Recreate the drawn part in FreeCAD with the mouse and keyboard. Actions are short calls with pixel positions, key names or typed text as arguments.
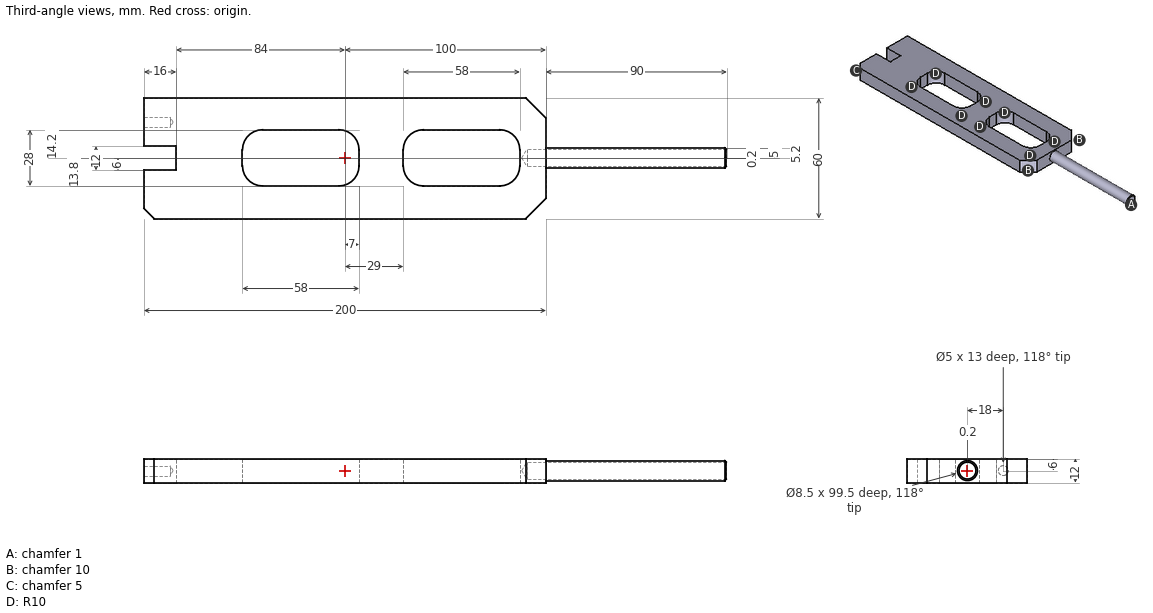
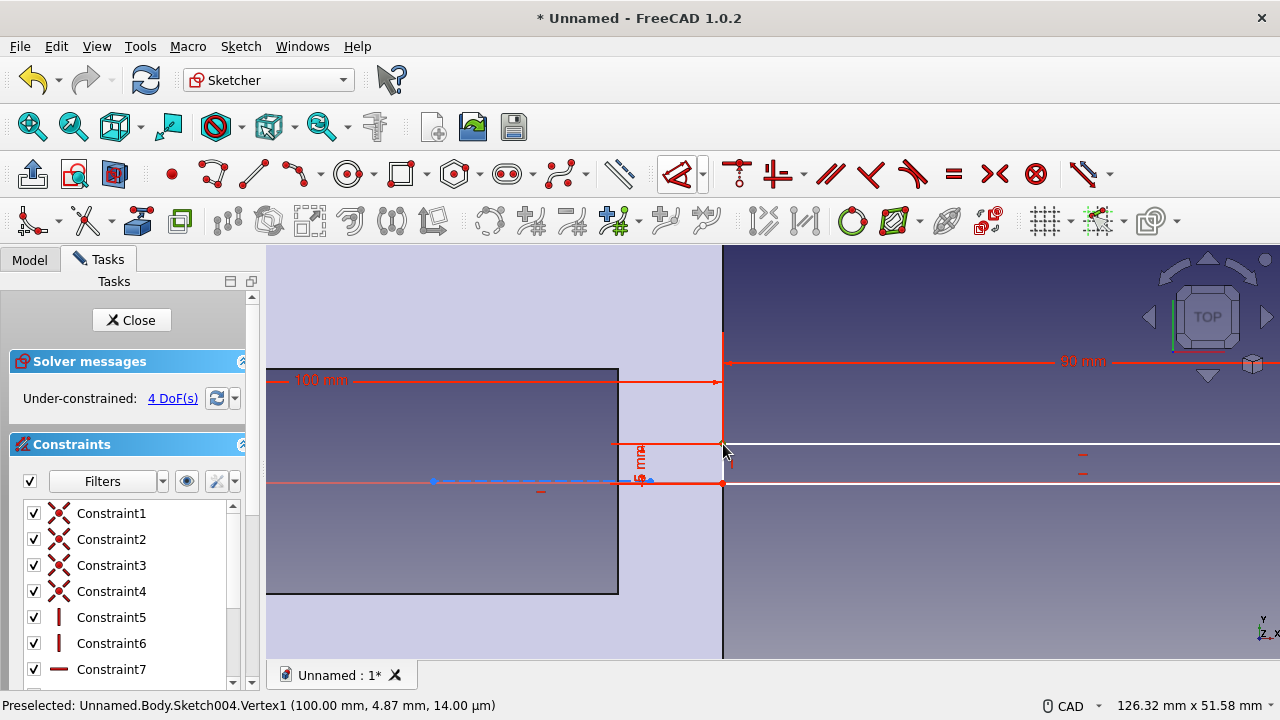
key(i)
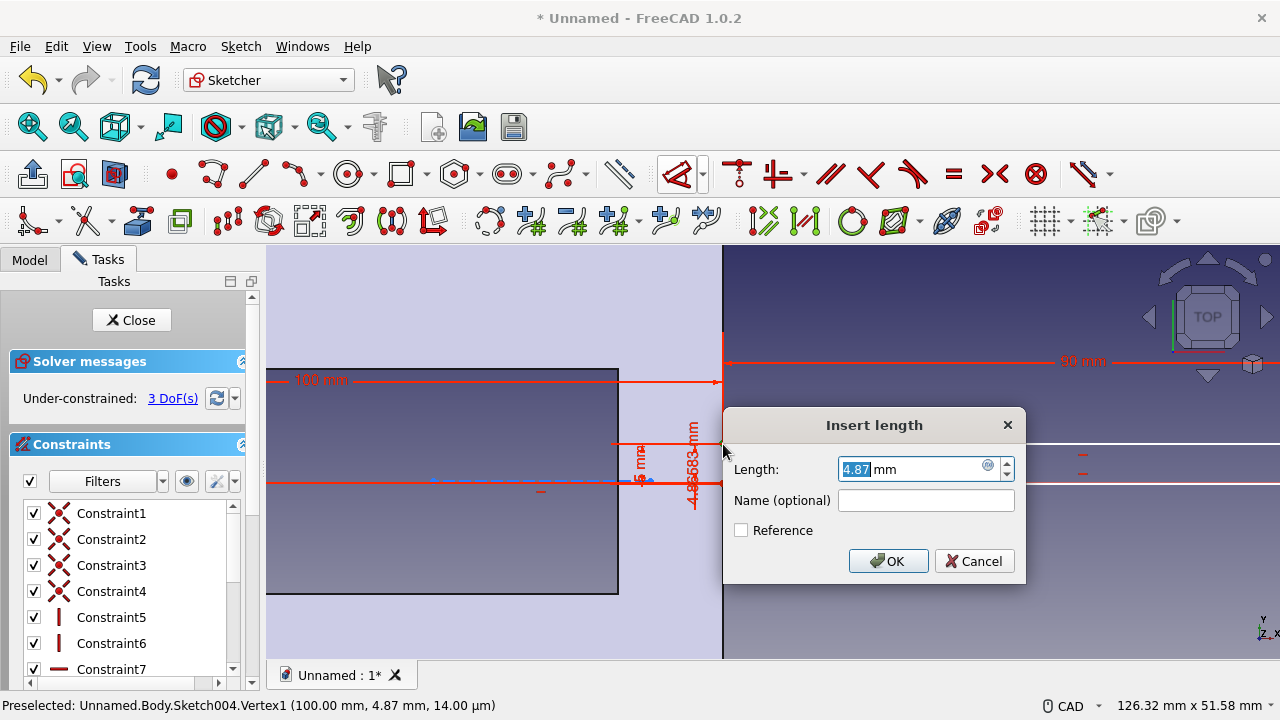
text(5.2)
key(Return)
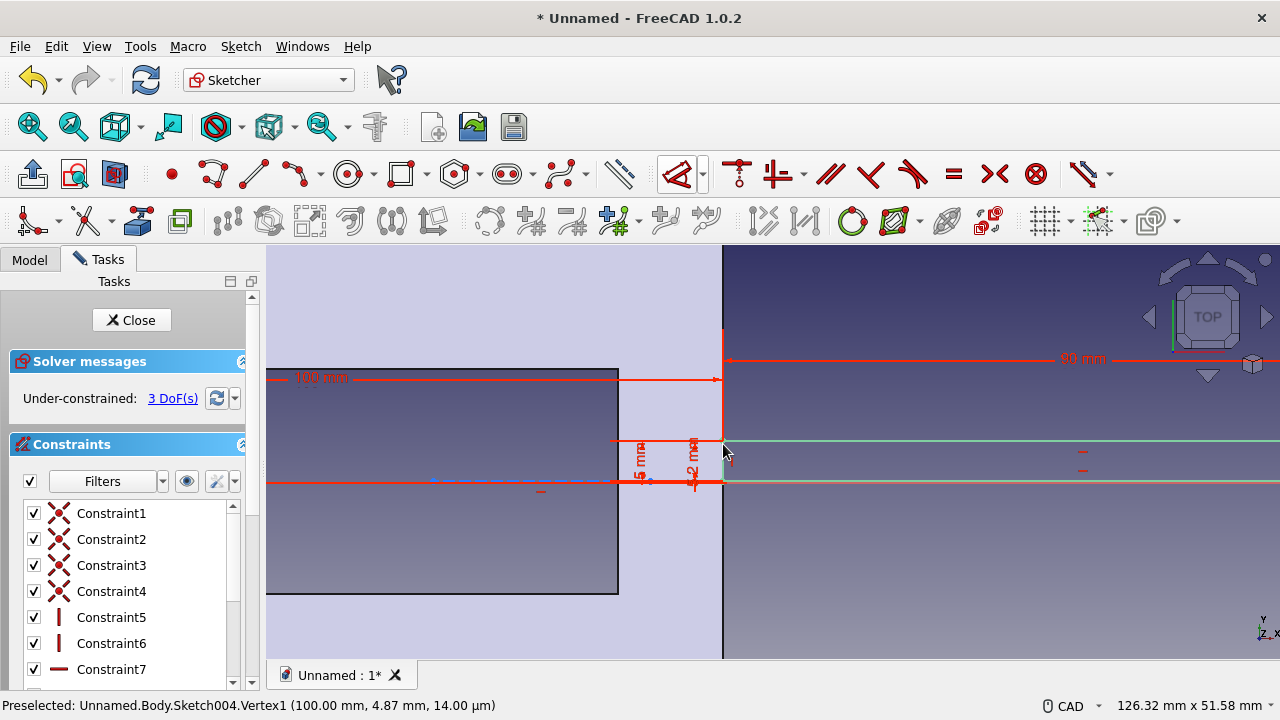
scroll(650, 481, up, 17)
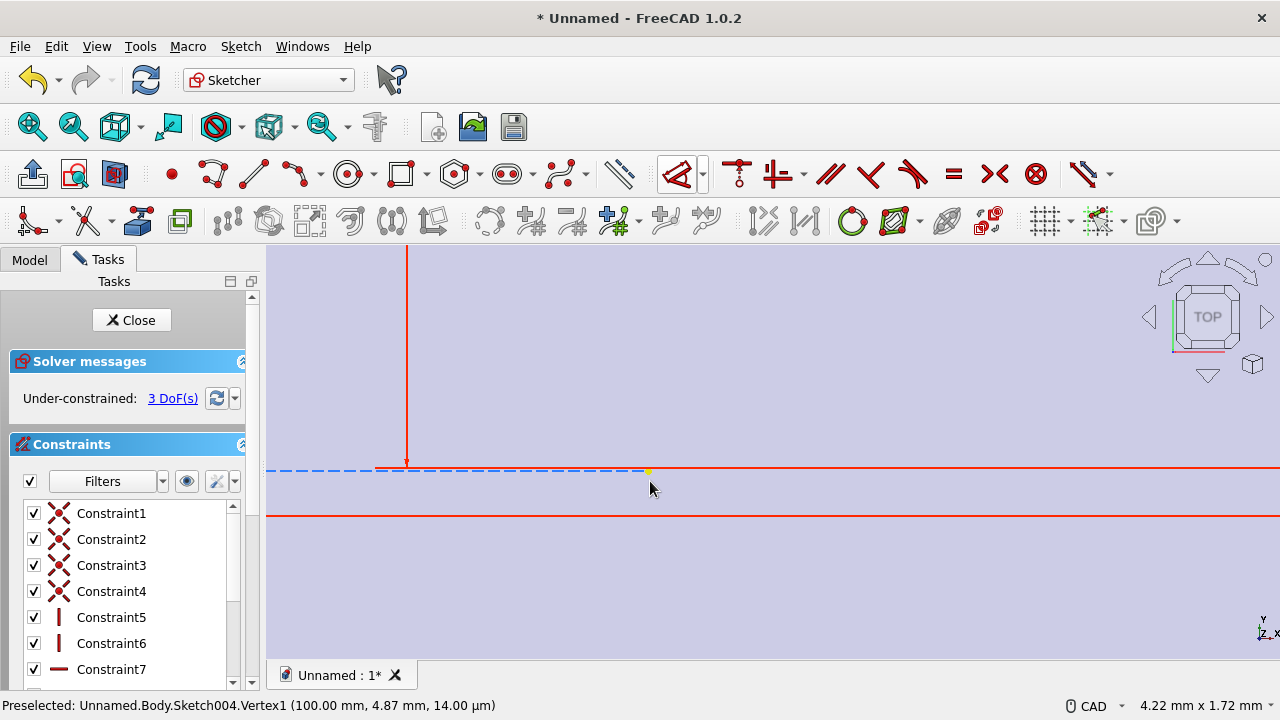
click(648, 471)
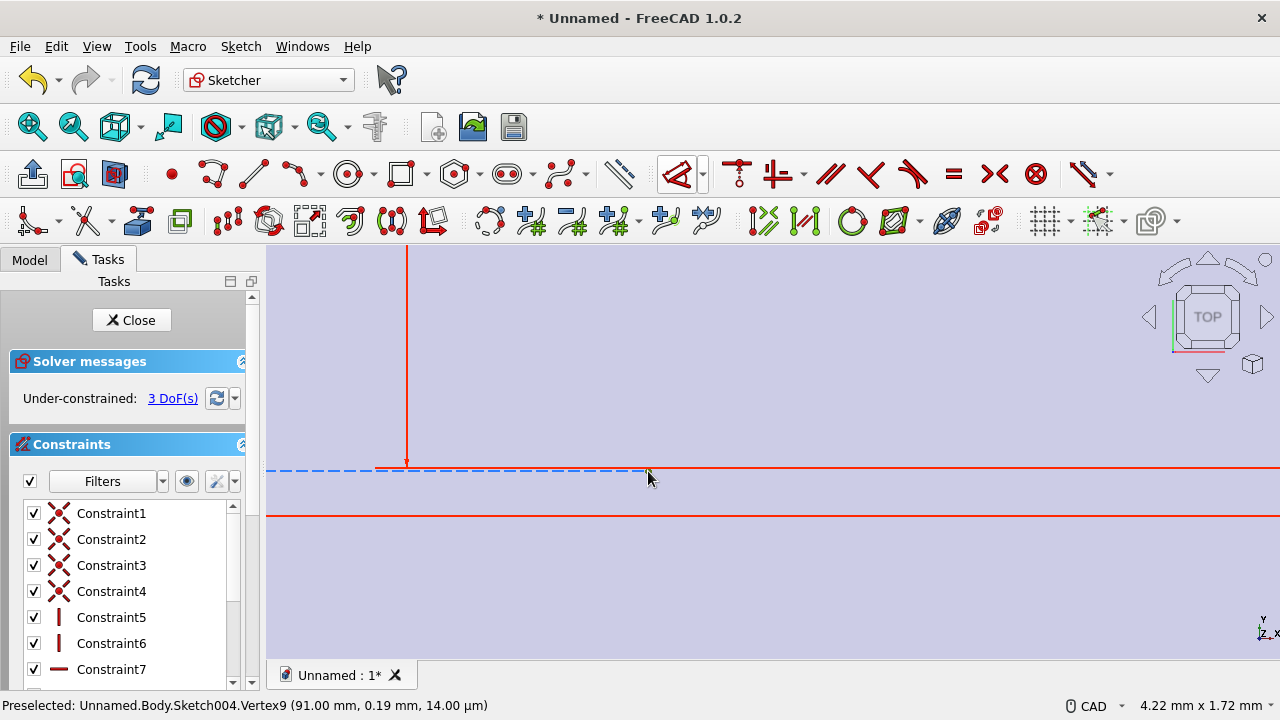
click(702, 174)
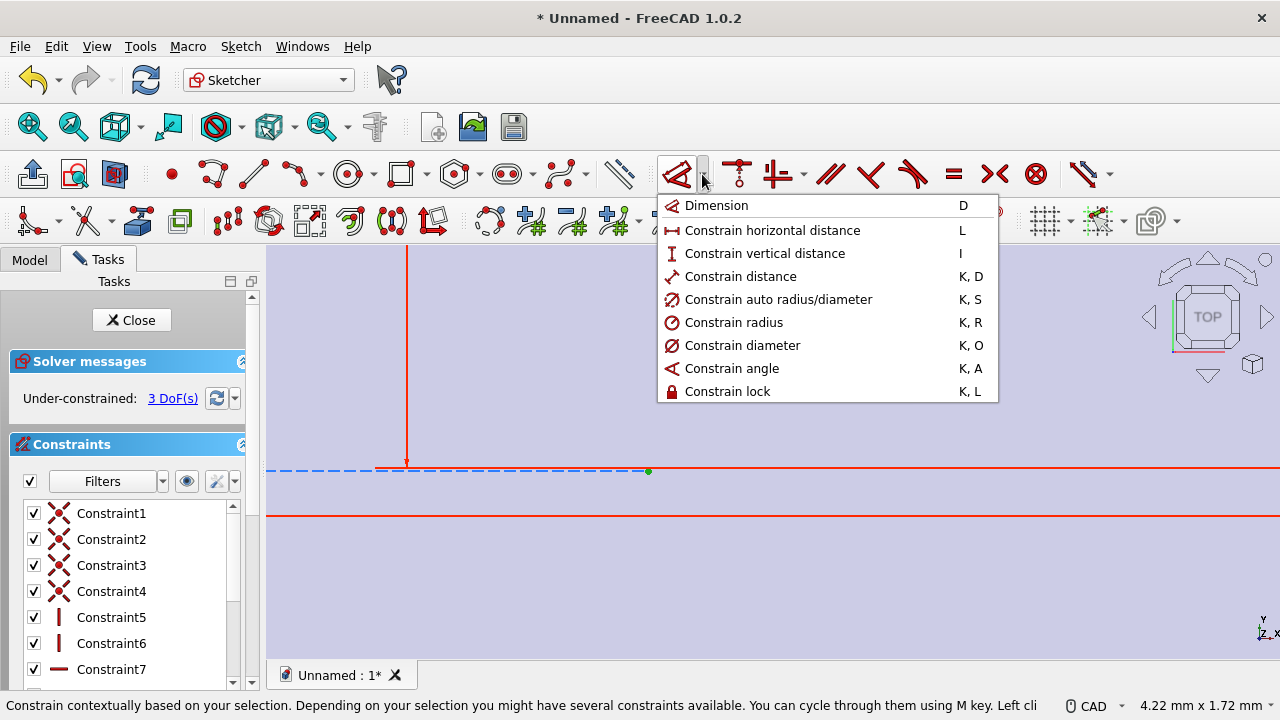
click(828, 254)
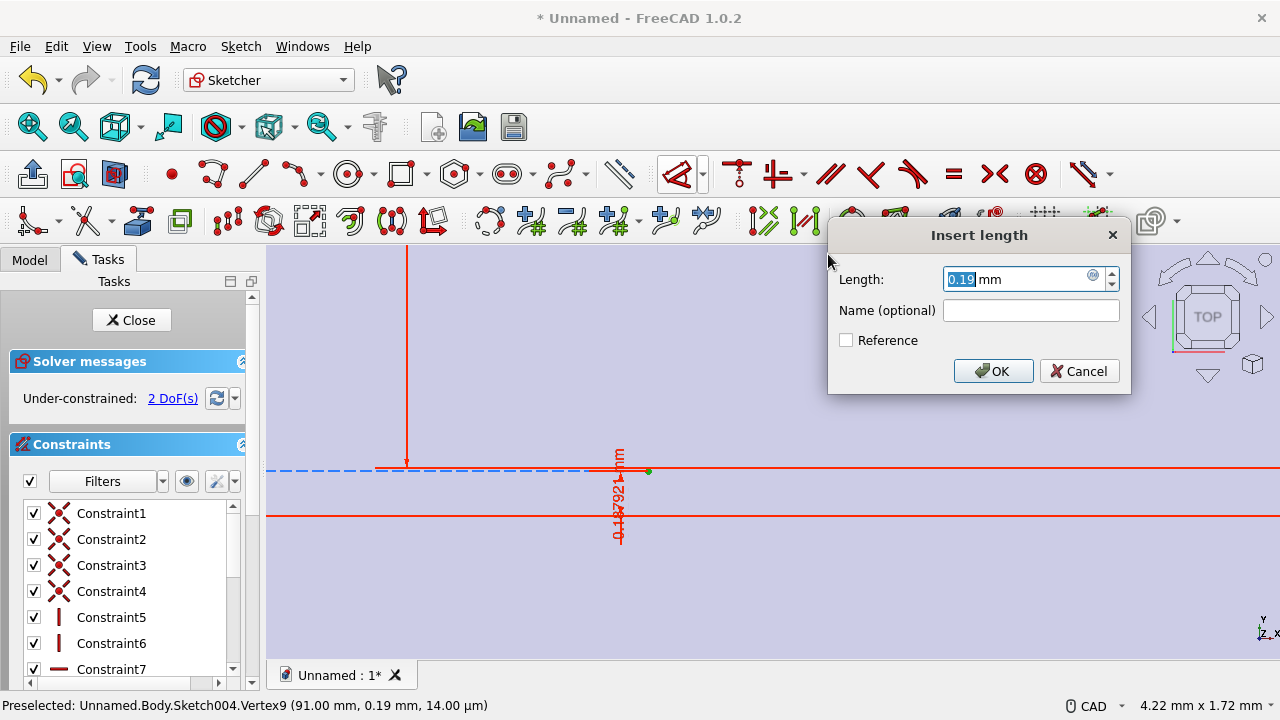
text(0.2)
key(Return)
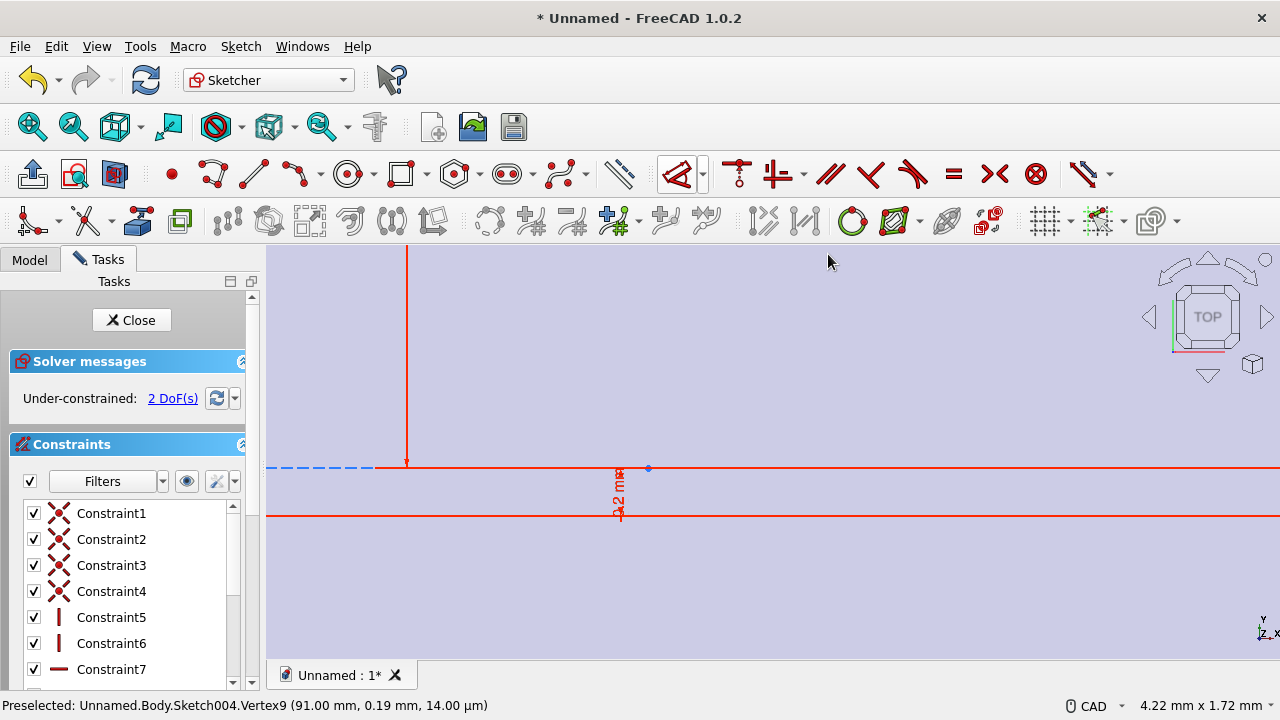
click(132, 320)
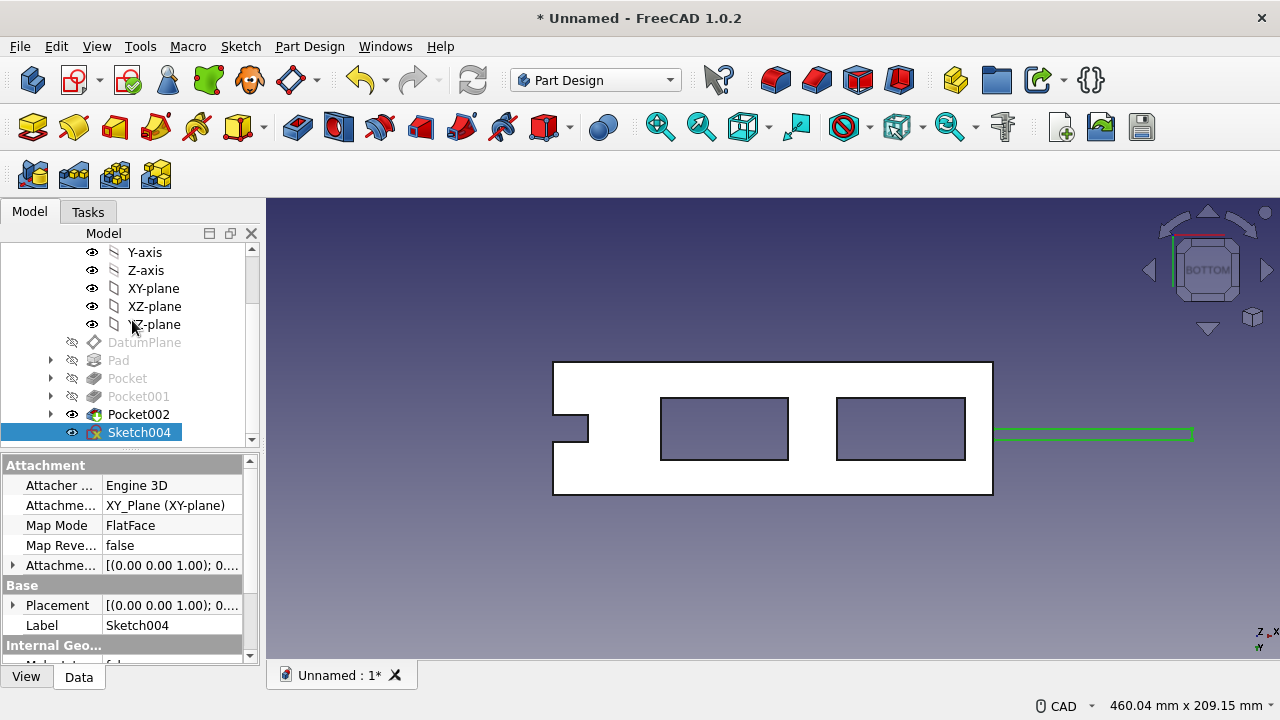
click(74, 128)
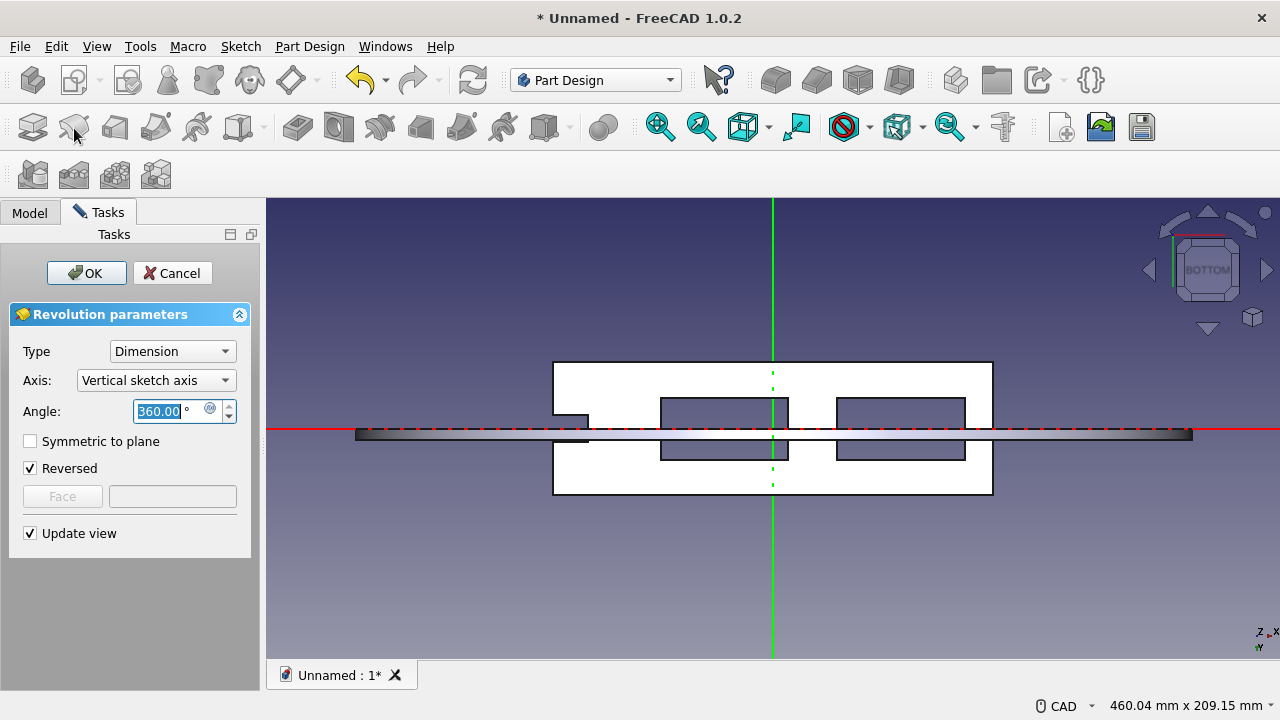
click(157, 380)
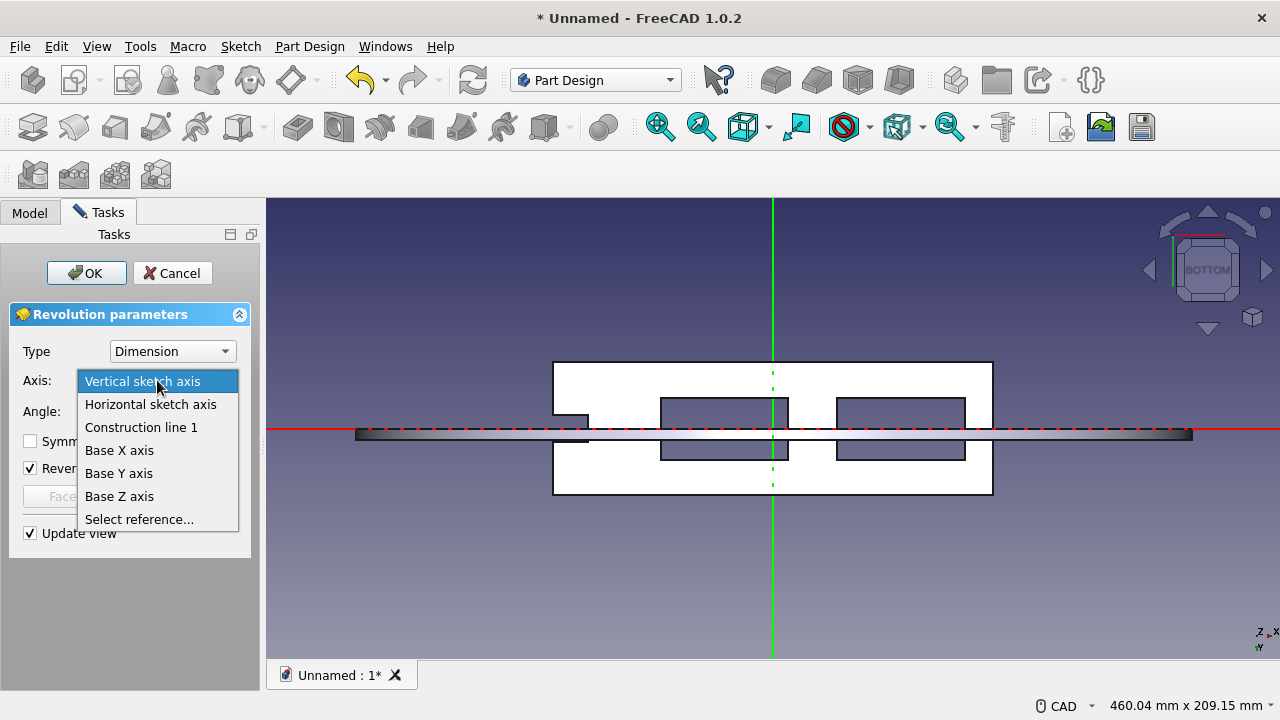
click(156, 428)